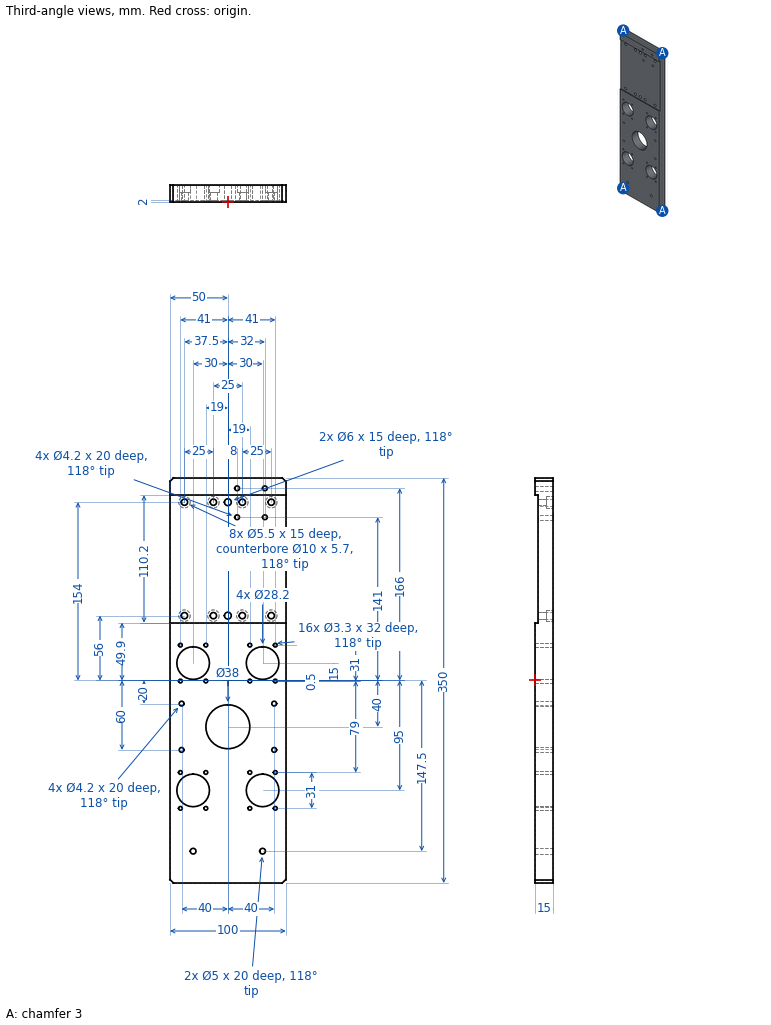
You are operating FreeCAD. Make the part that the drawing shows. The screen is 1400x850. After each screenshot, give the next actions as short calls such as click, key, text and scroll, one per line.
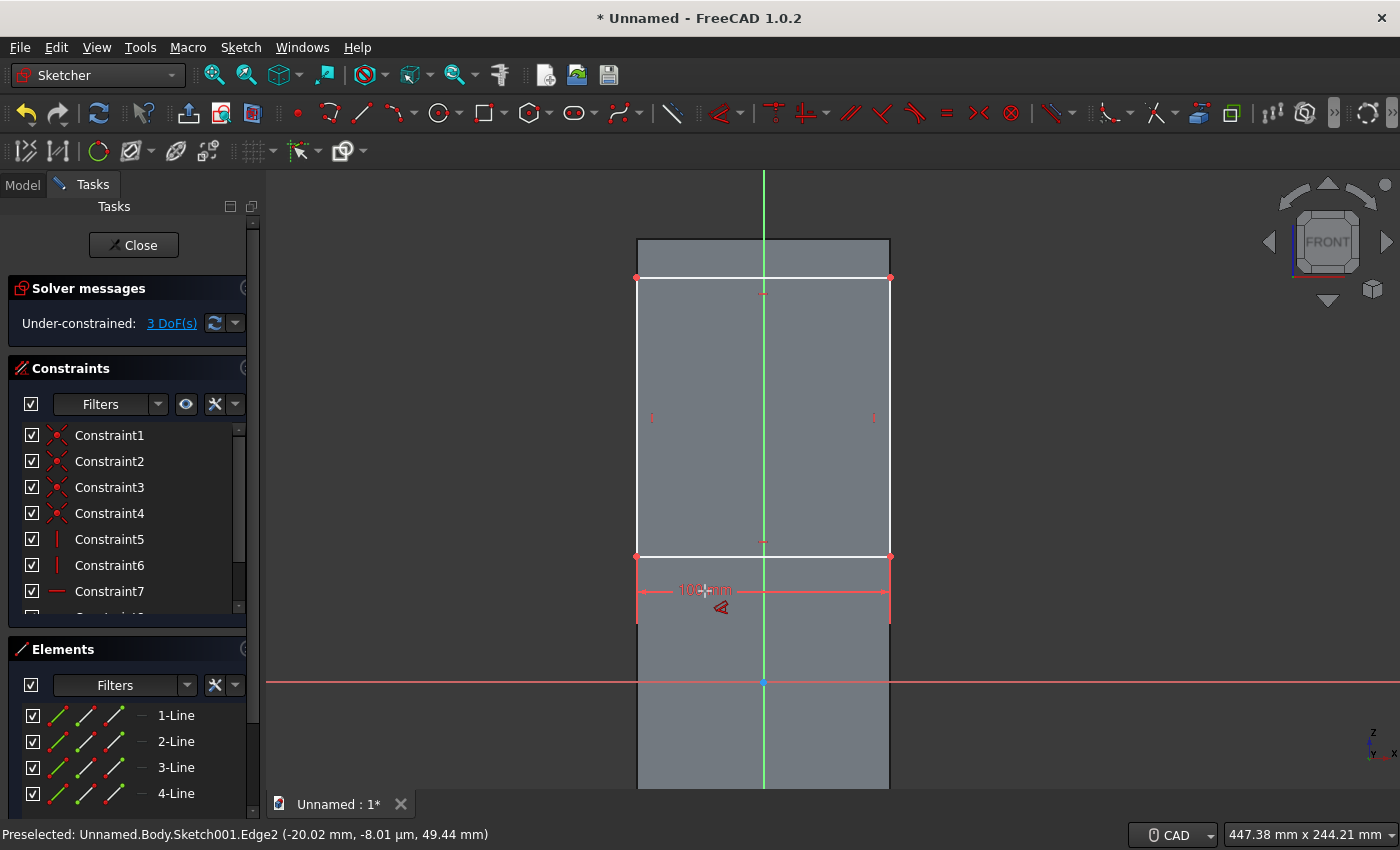
click(637, 278)
click(700, 716)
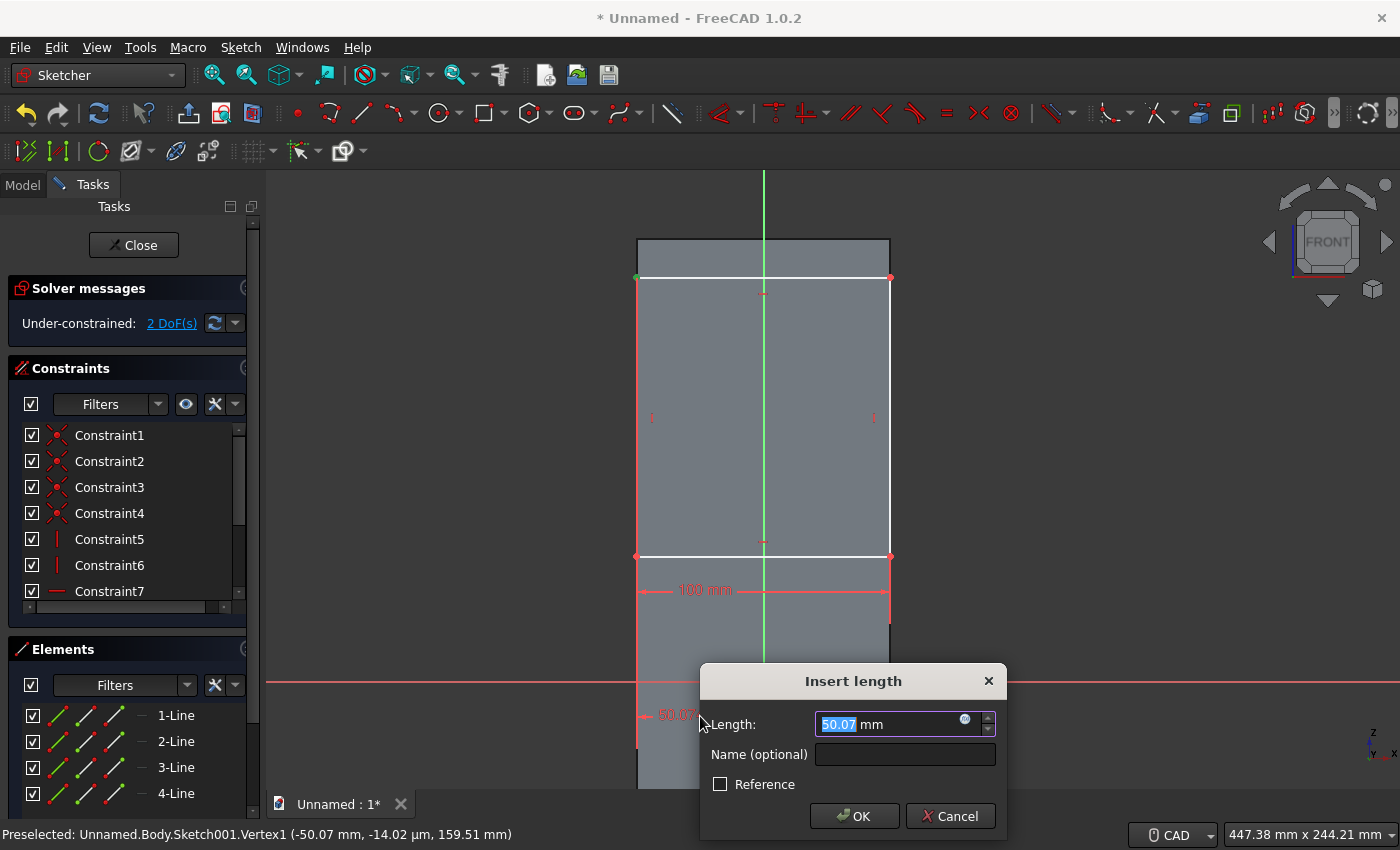
text(50)
key(Return)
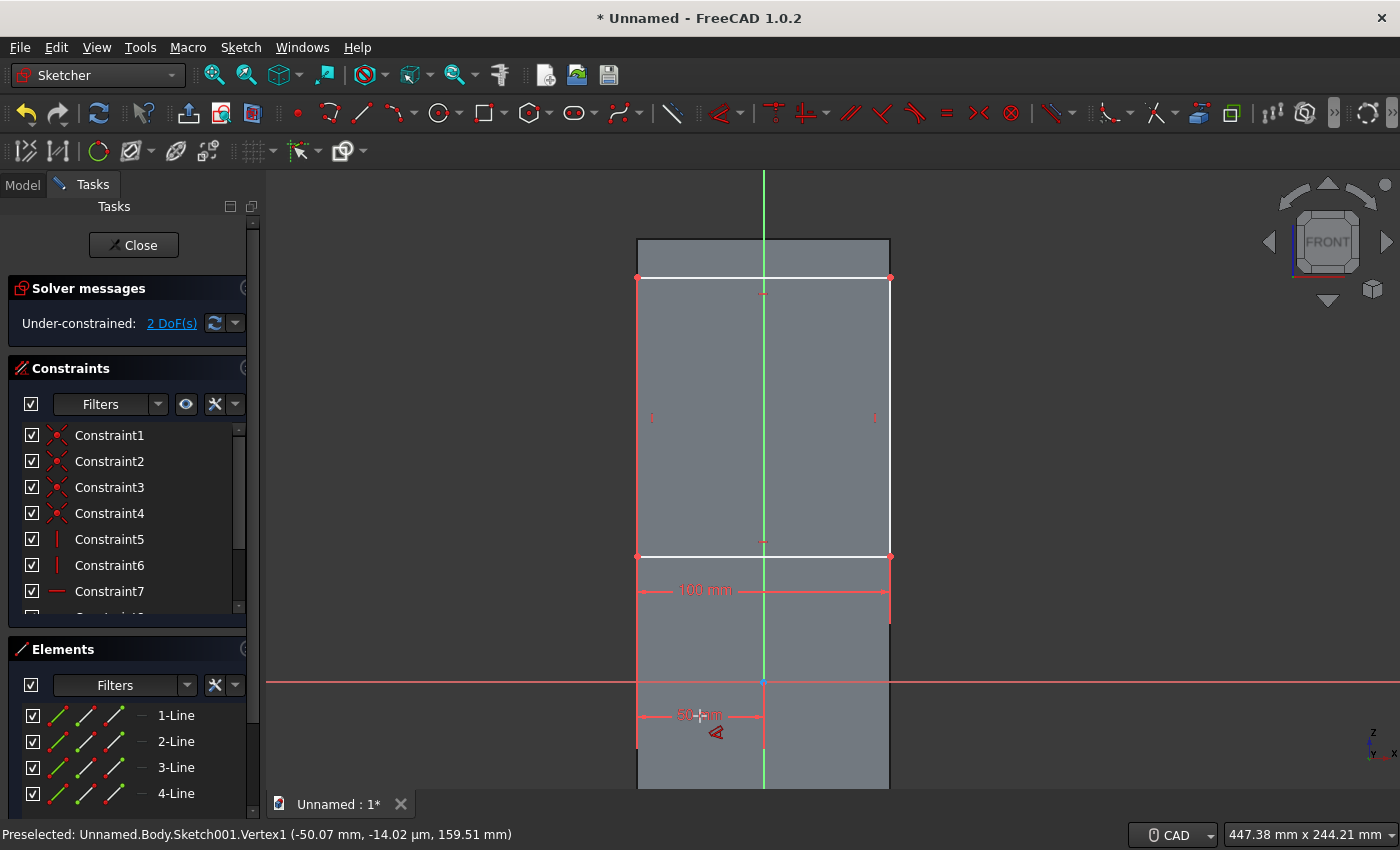
click(637, 362)
click(603, 417)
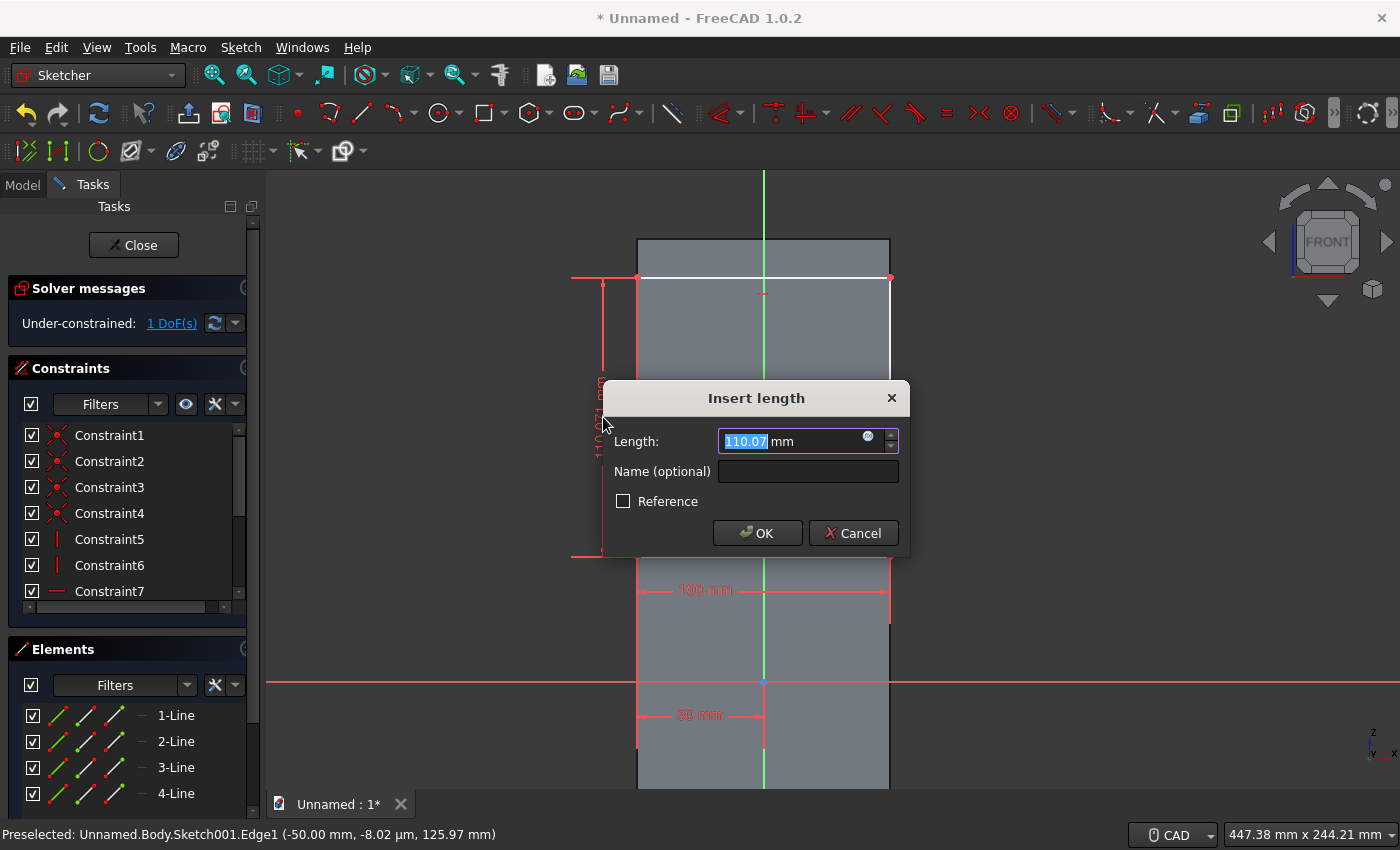
text(110.2)
key(Return)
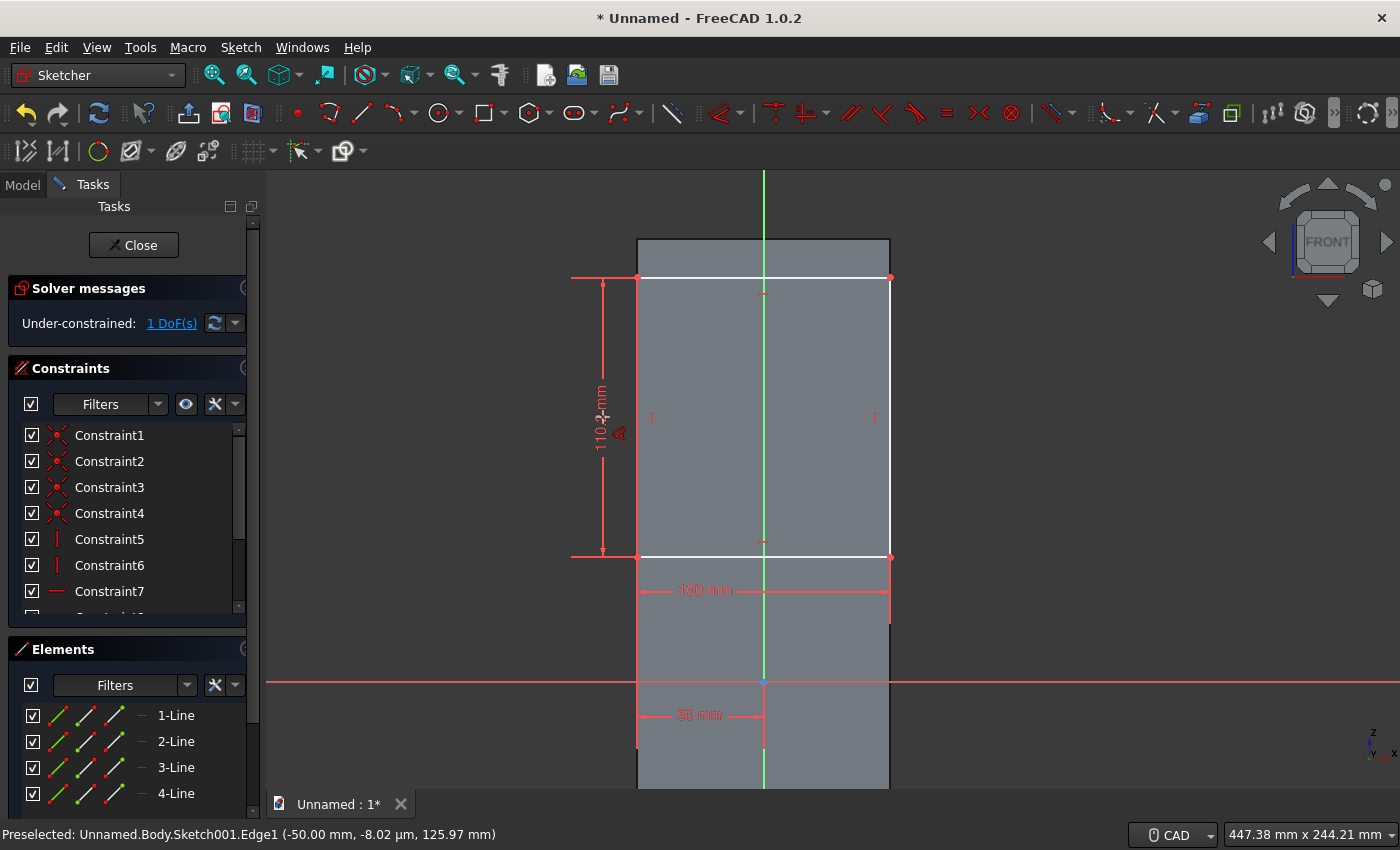
click(637, 557)
click(603, 620)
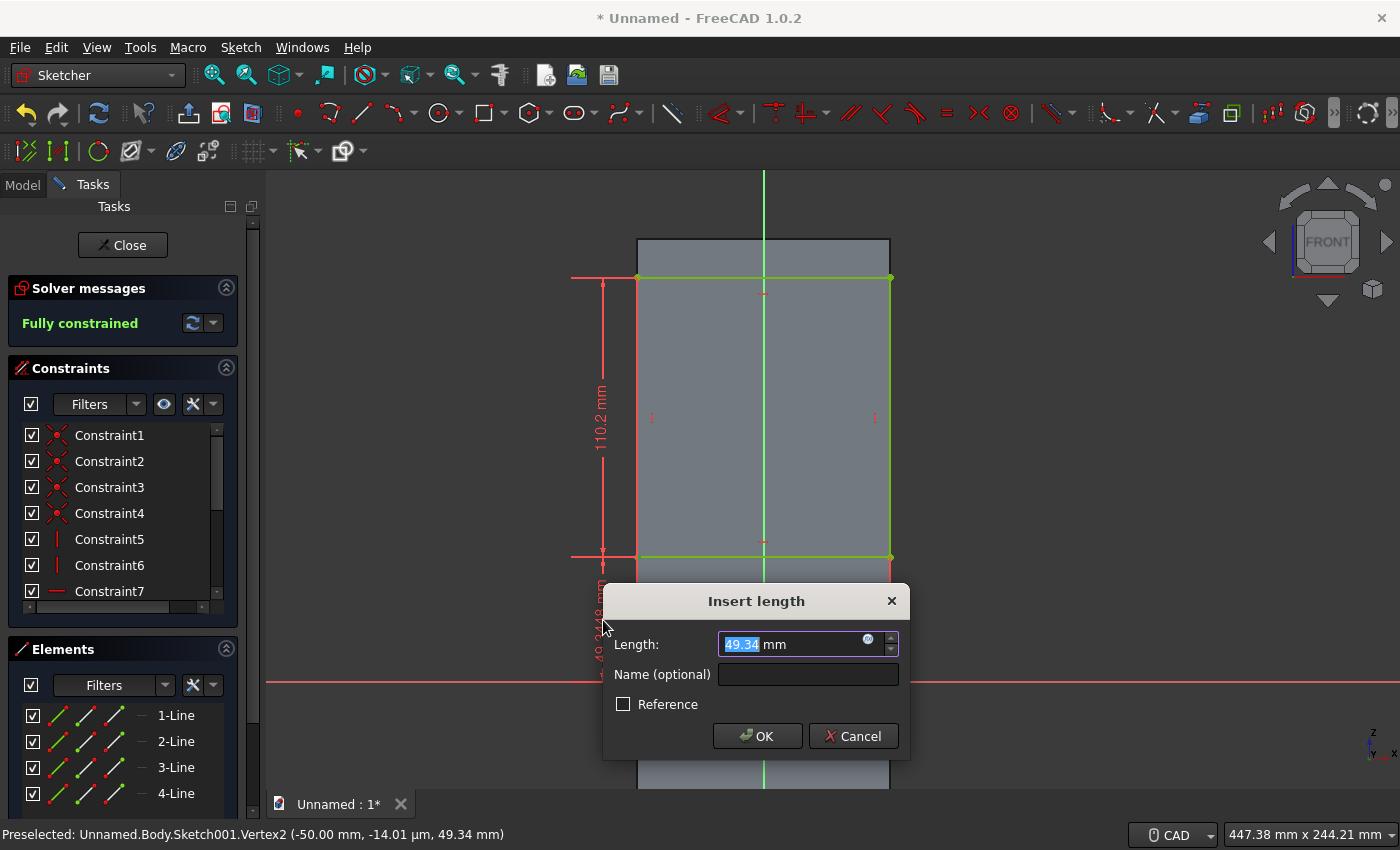
text(49.9)
key(Return)
key(Escape)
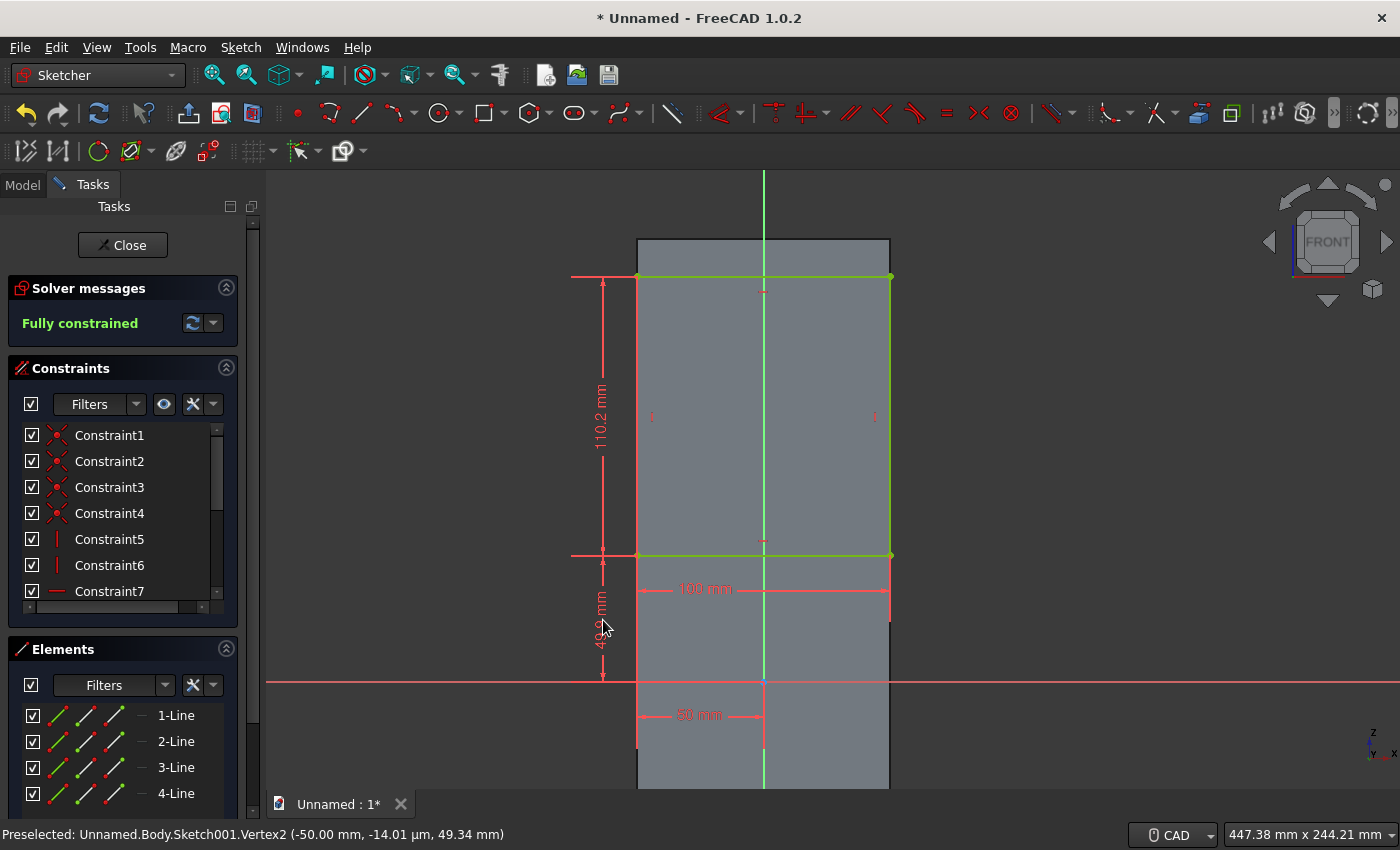
click(123, 245)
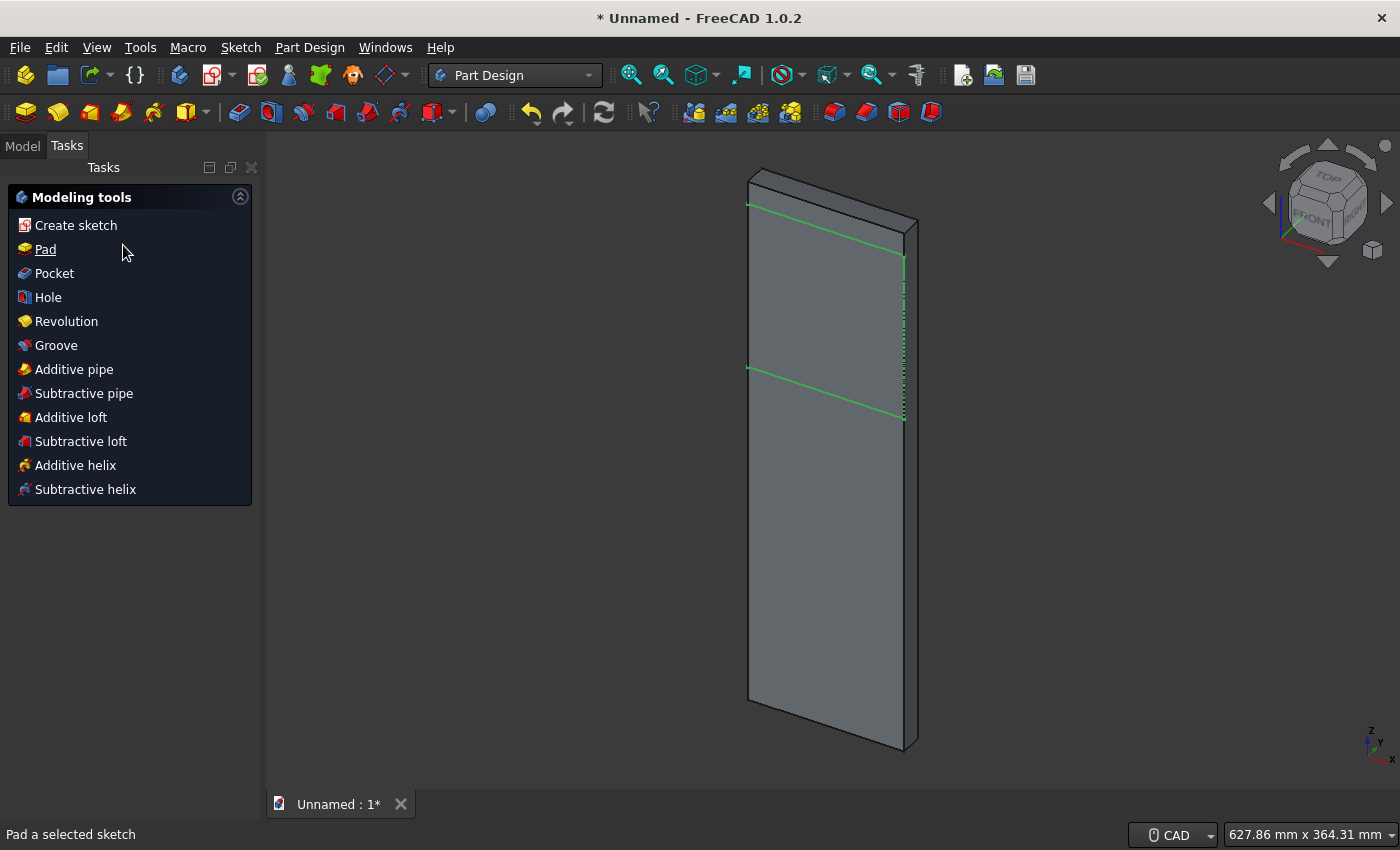
click(240, 112)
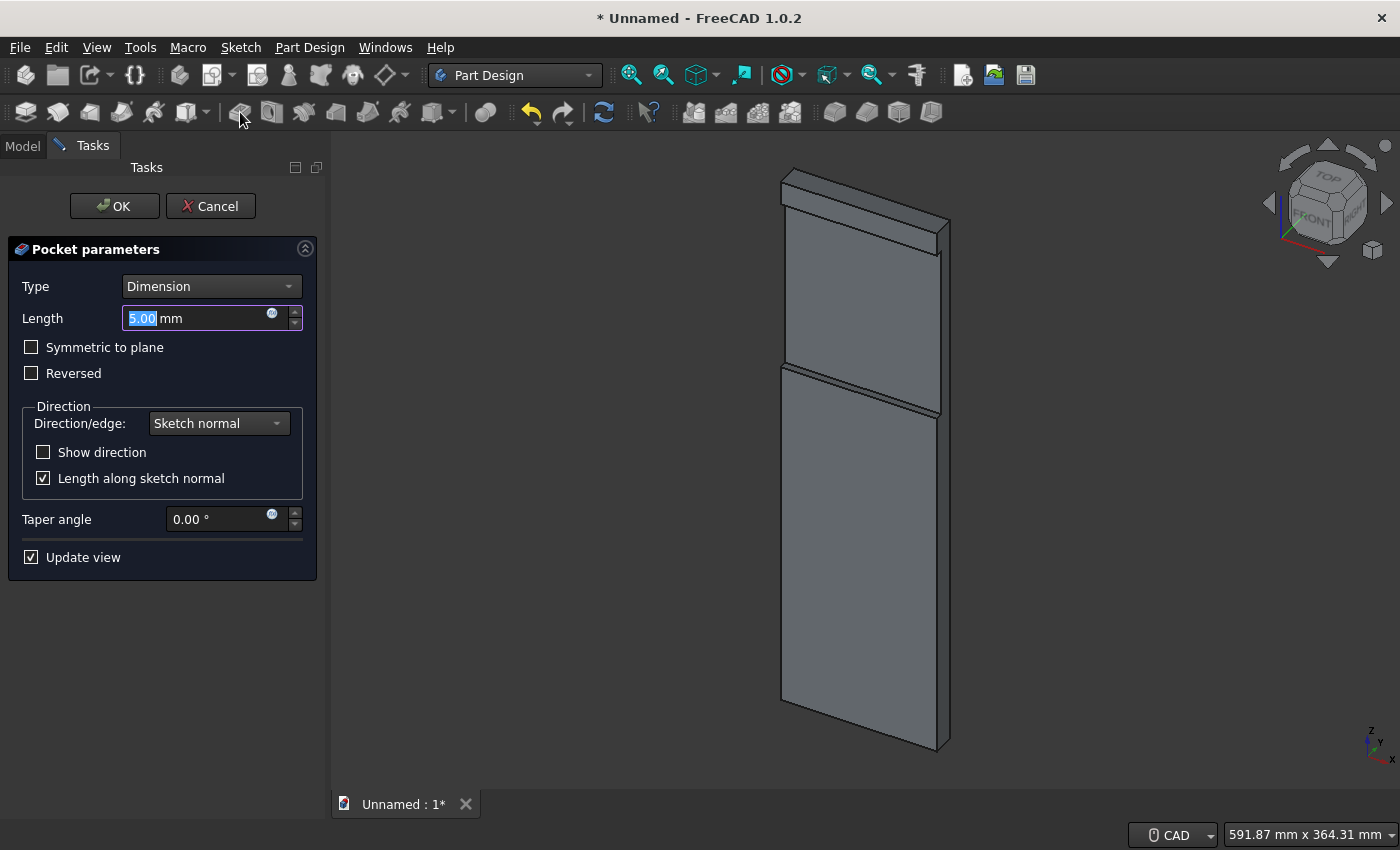
text(2)
key(Tab)